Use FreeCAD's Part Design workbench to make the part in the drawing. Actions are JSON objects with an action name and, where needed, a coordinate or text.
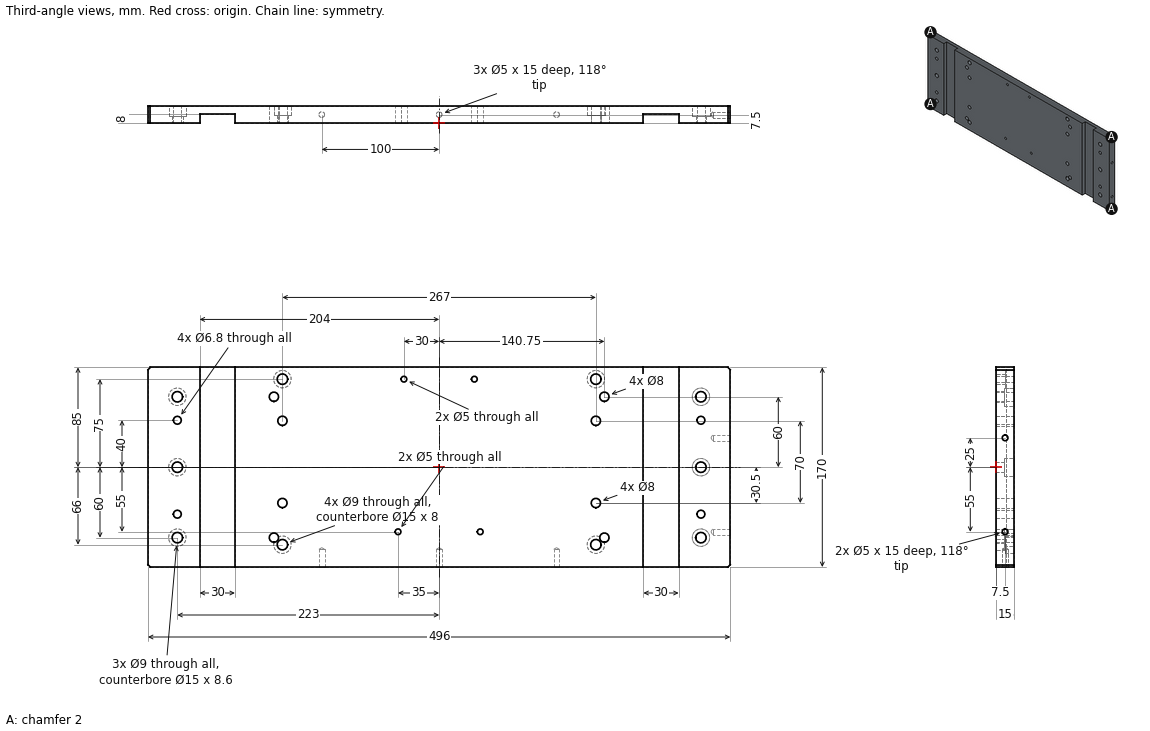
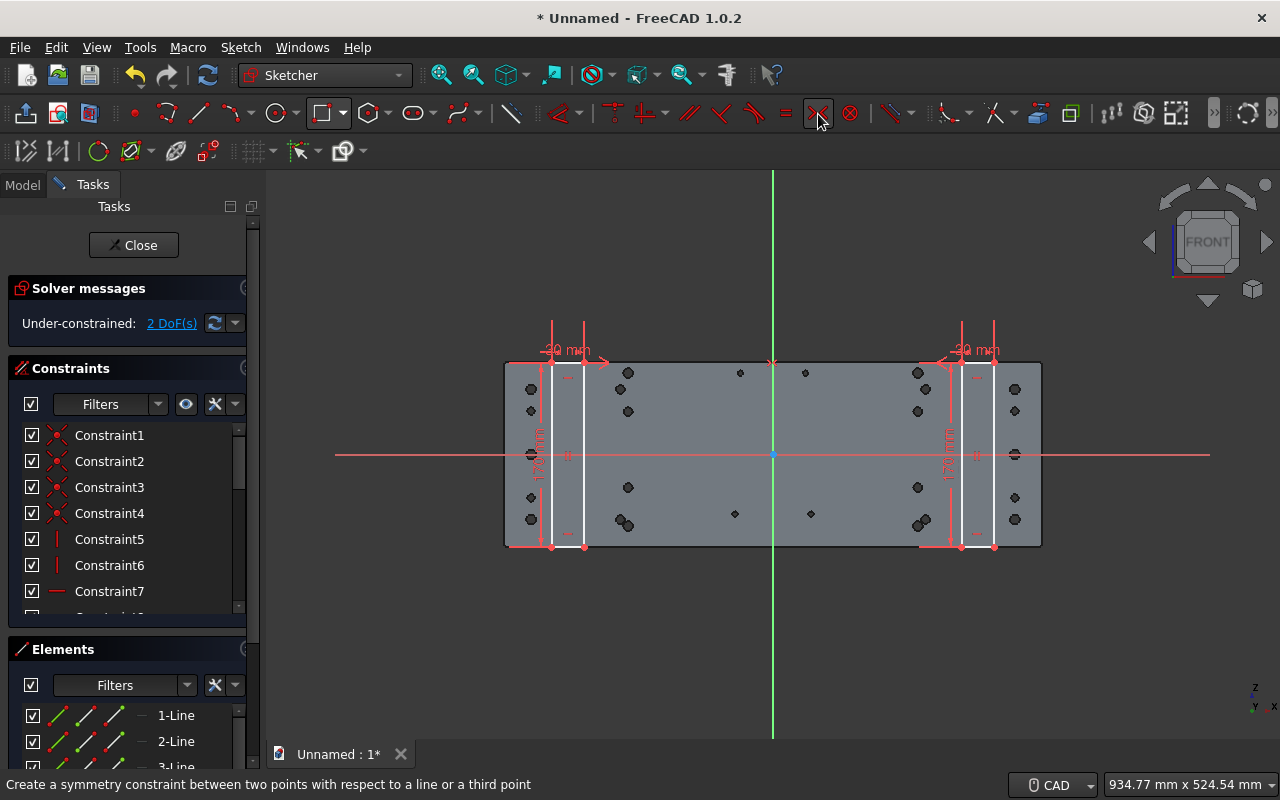
{"action": "left_click", "coordinate": [558, 114]}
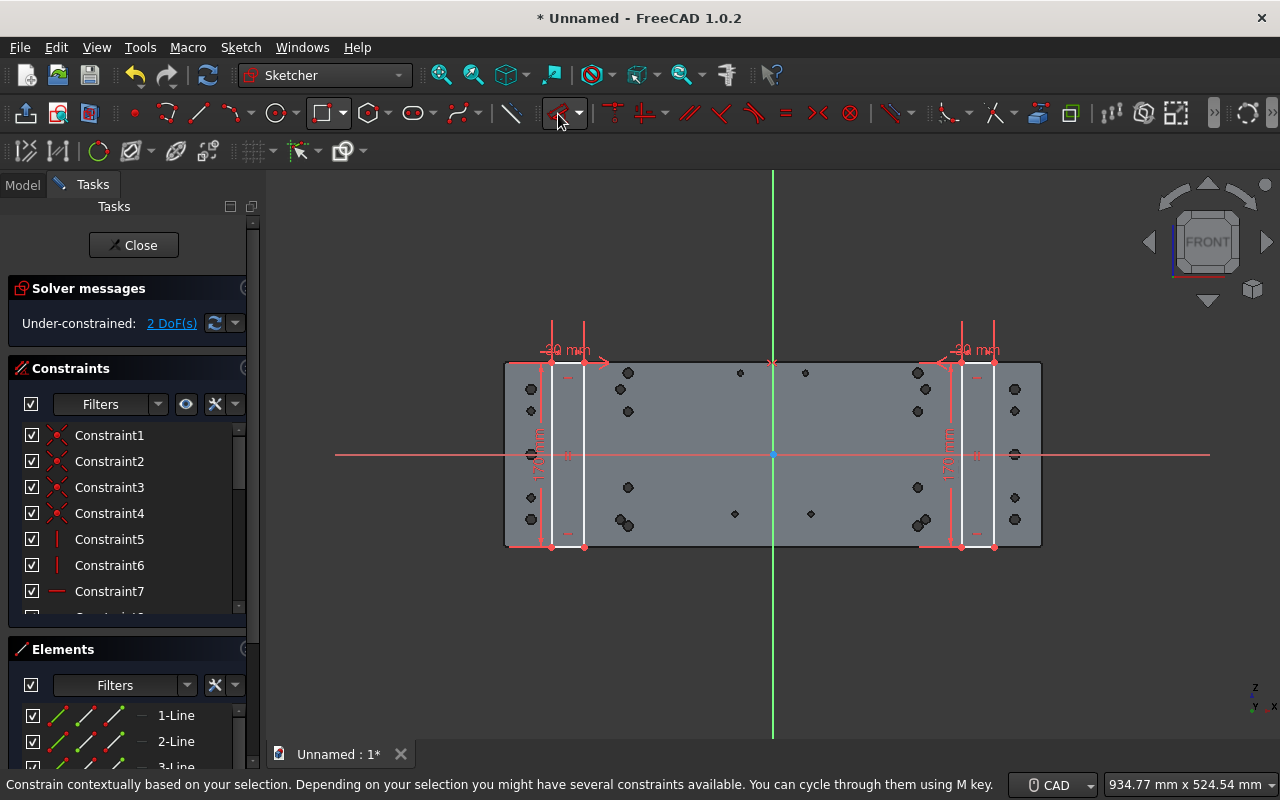
{"action": "left_click", "coordinate": [552, 363]}
{"action": "left_click", "coordinate": [518, 409]}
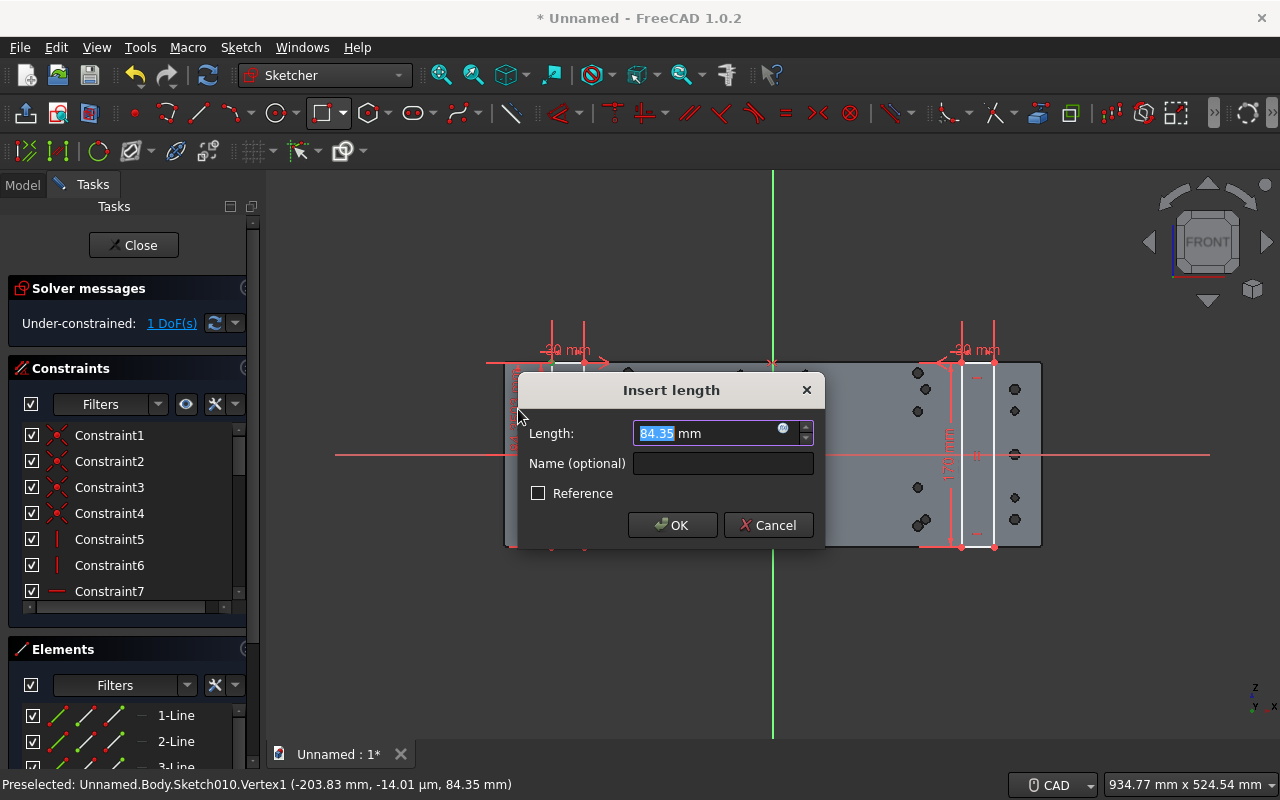
{"action": "type", "text": "85"}
{"action": "key", "text": "Return"}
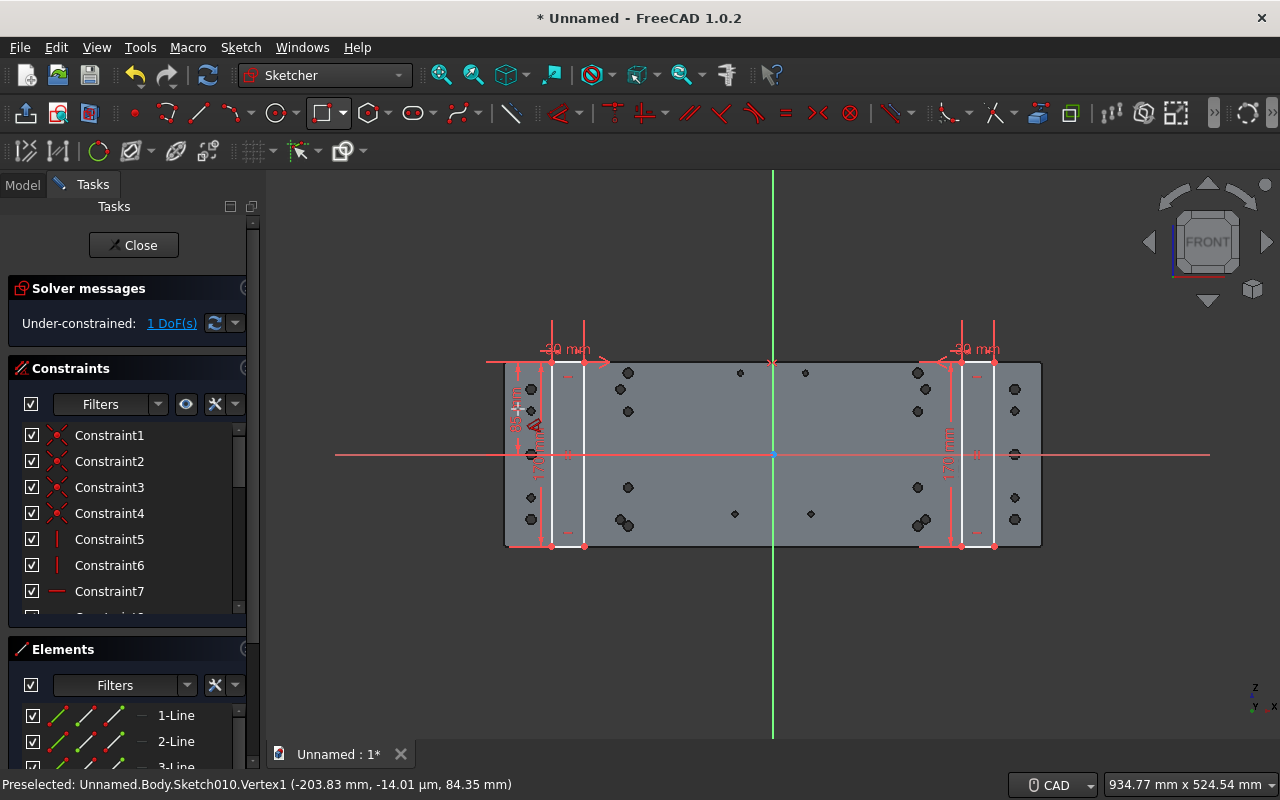
{"action": "left_click", "coordinate": [552, 362]}
{"action": "left_click", "coordinate": [662, 328]}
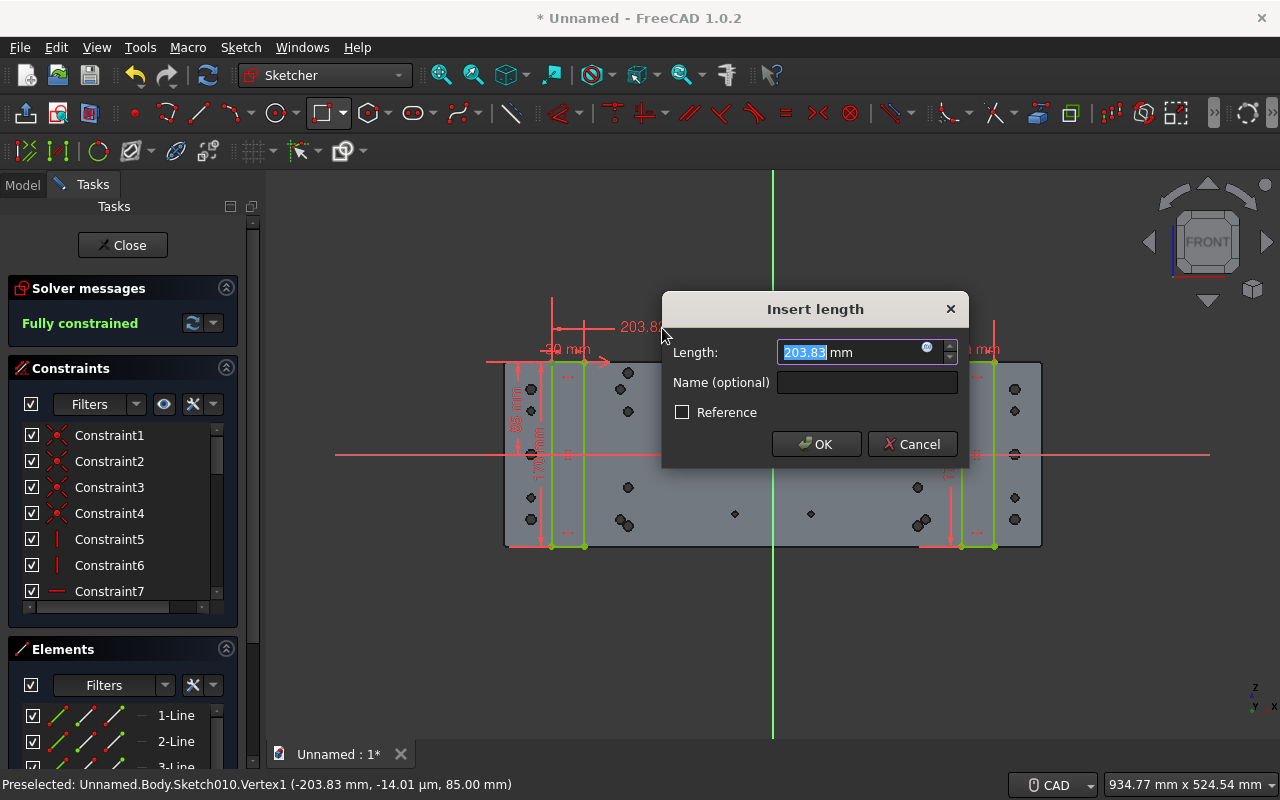
{"action": "type", "text": "204"}
{"action": "key", "text": "Return"}
{"action": "key", "text": "Escape"}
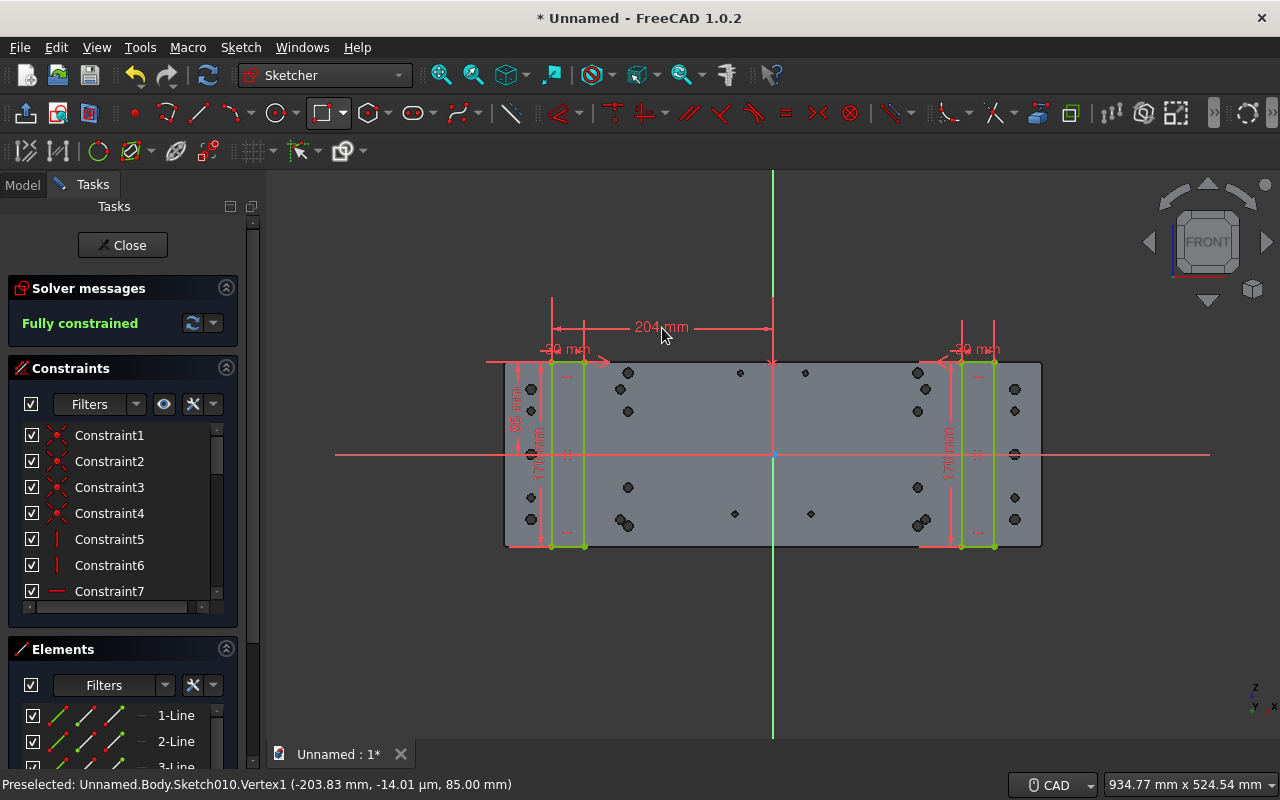
{"action": "left_click", "coordinate": [123, 245]}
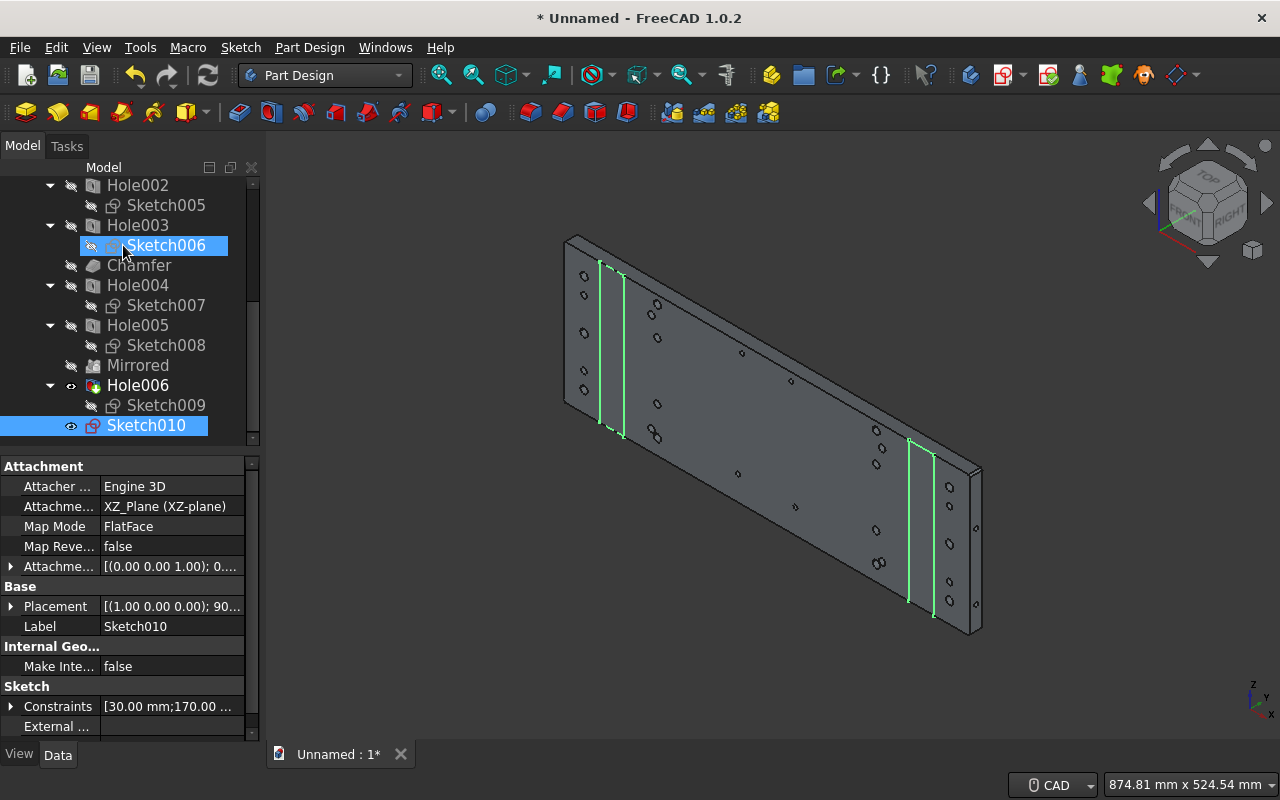
{"action": "left_click", "coordinate": [240, 112]}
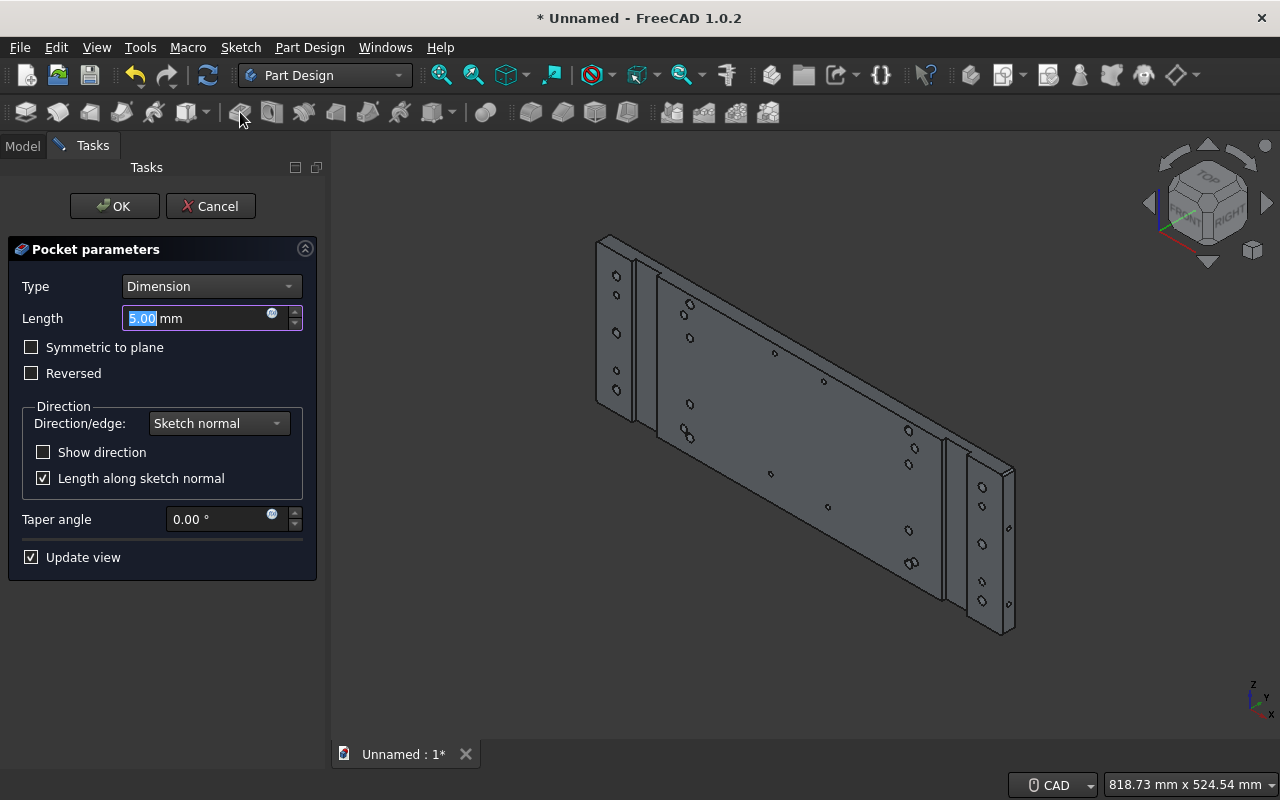
{"action": "type", "text": "8"}
{"action": "key", "text": "Tab"}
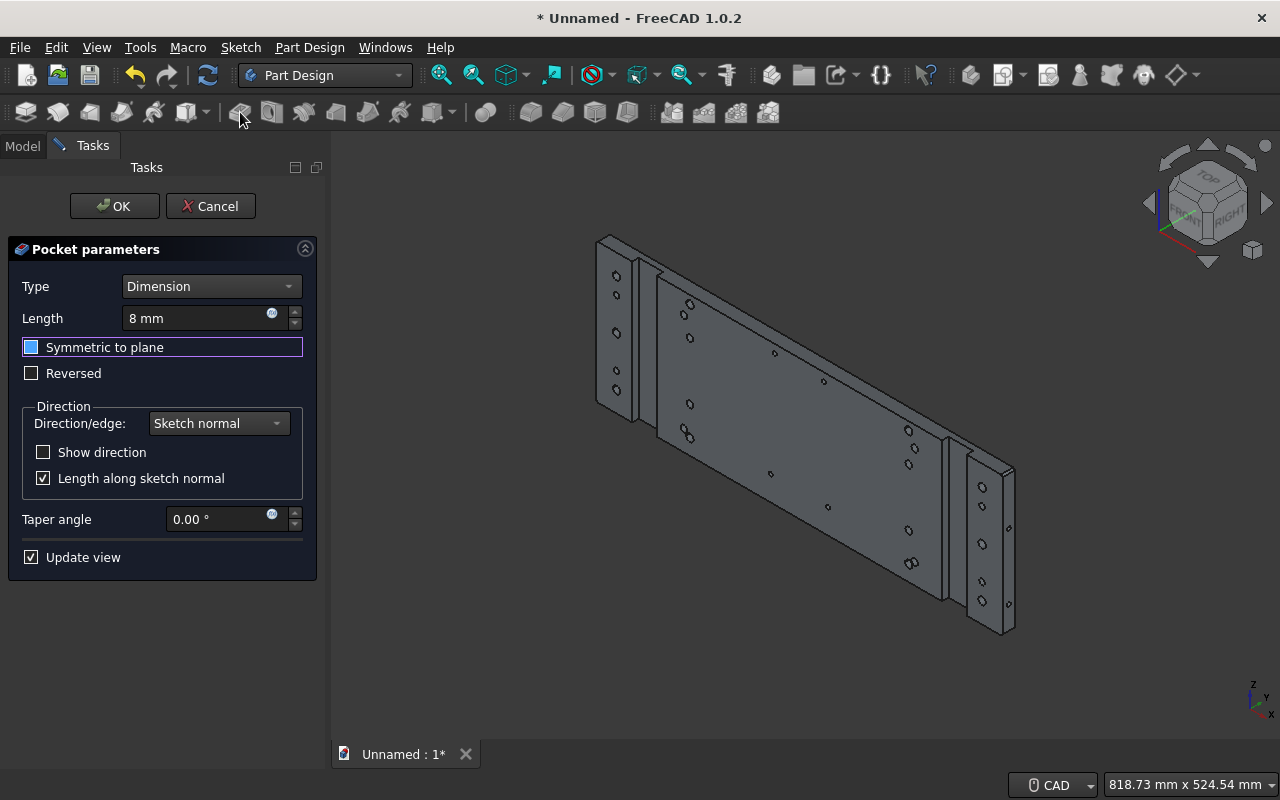
{"action": "left_click", "coordinate": [115, 206]}